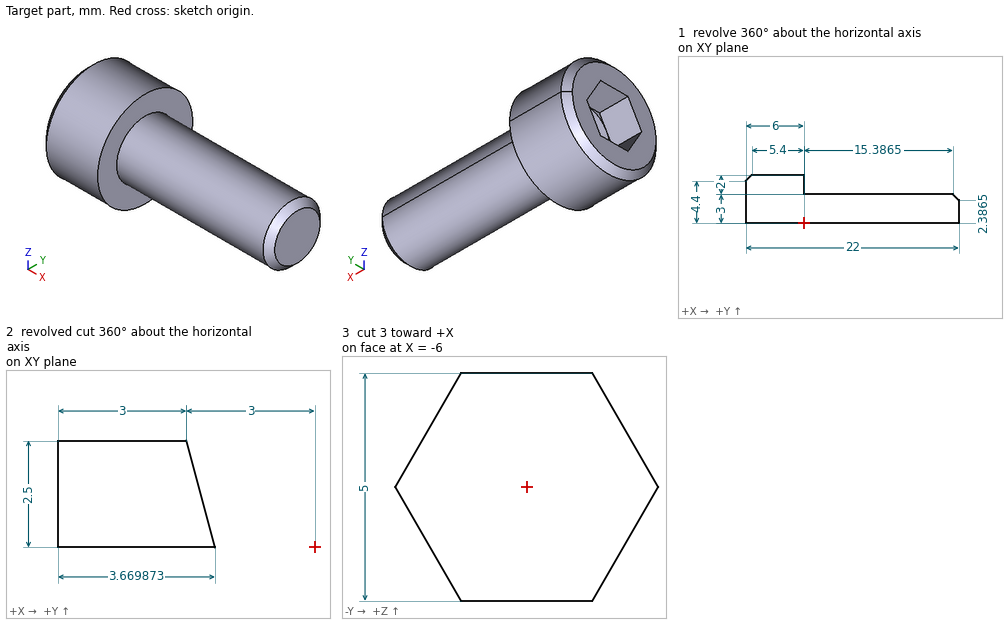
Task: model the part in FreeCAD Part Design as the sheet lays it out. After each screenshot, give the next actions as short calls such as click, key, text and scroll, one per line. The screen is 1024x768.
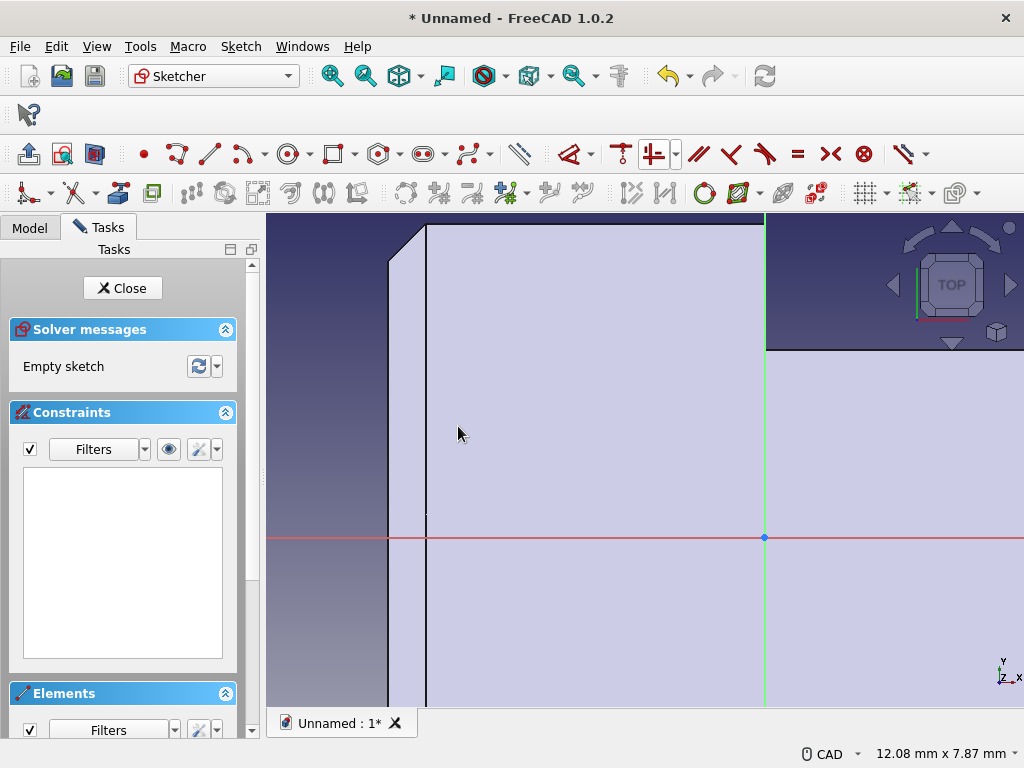
click(177, 154)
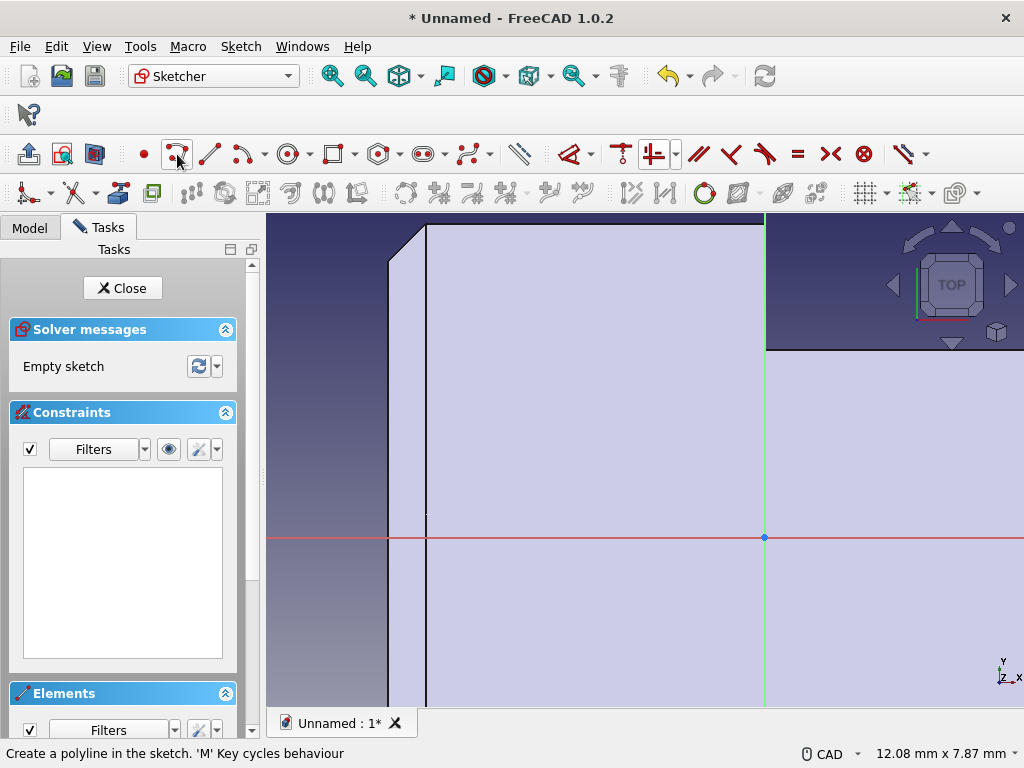
click(618, 538)
click(576, 381)
click(388, 381)
click(388, 529)
click(618, 538)
key(Escape)
key(Escape)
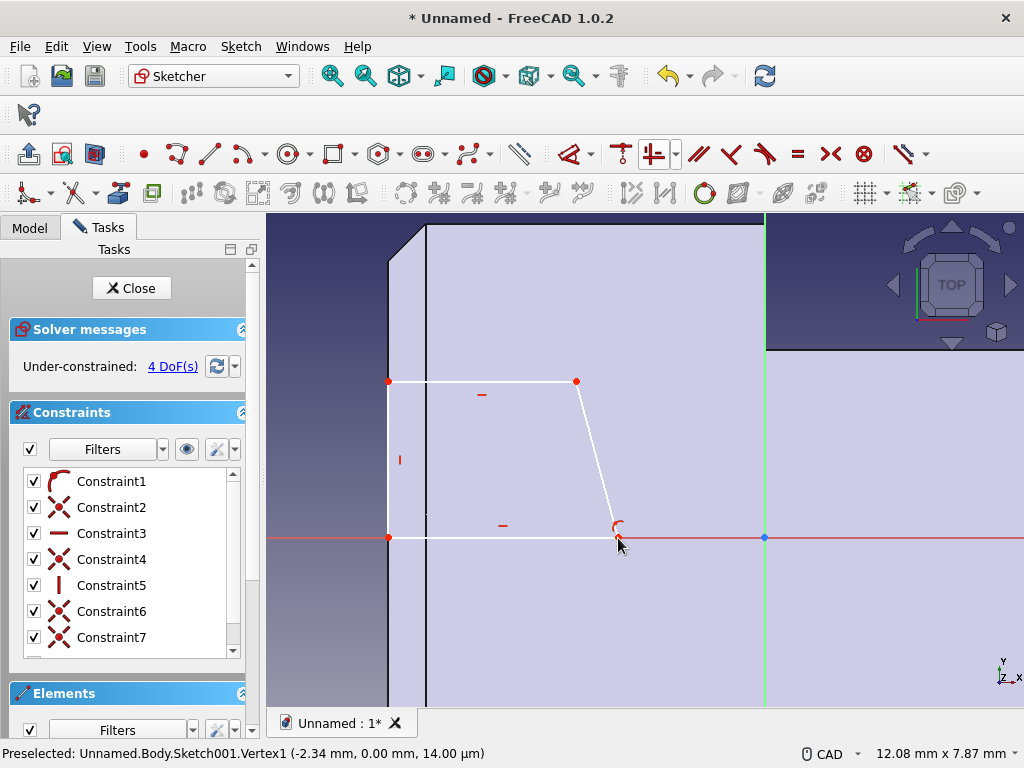
click(568, 154)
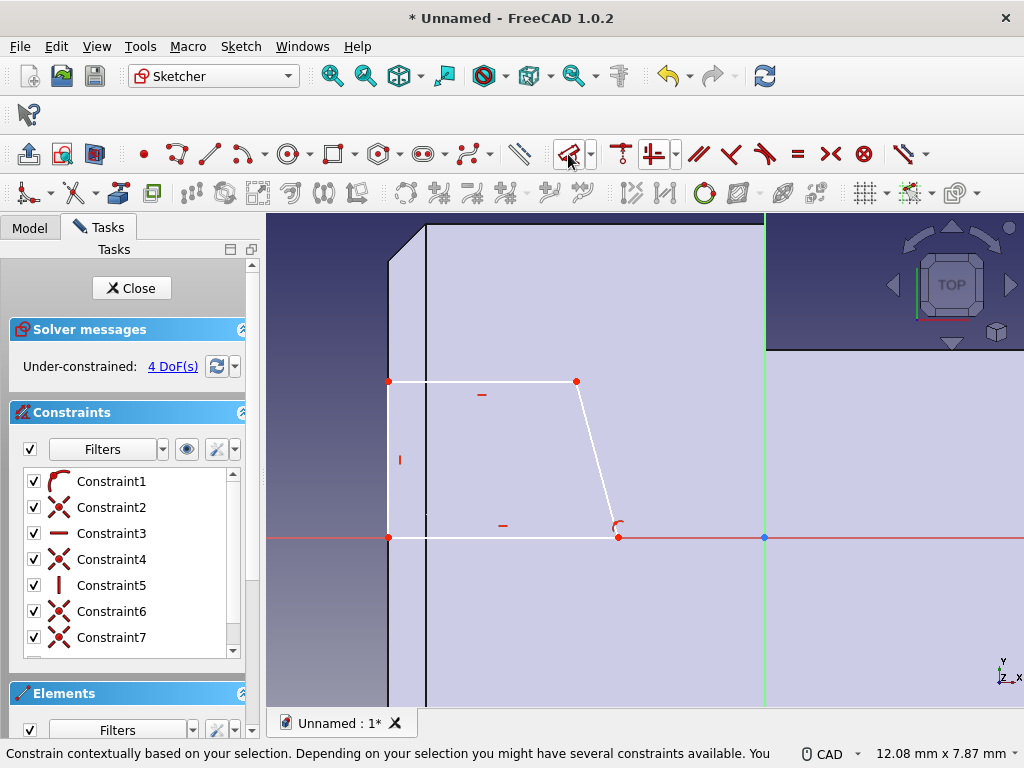
click(520, 382)
click(482, 348)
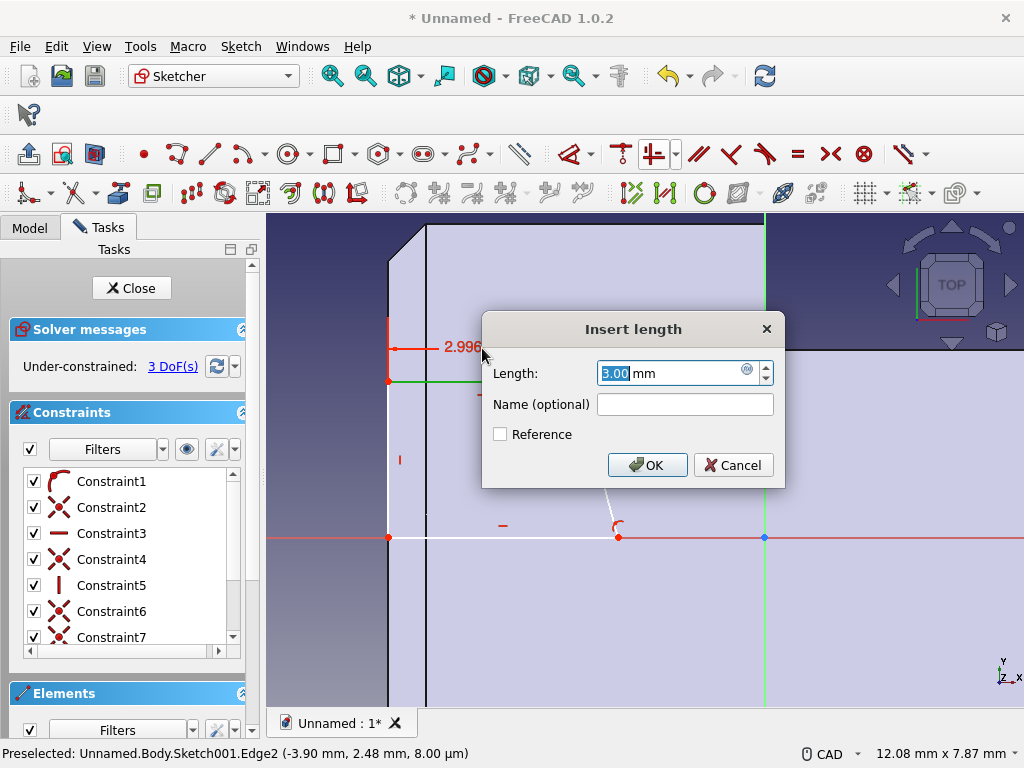
text(3)
key(Return)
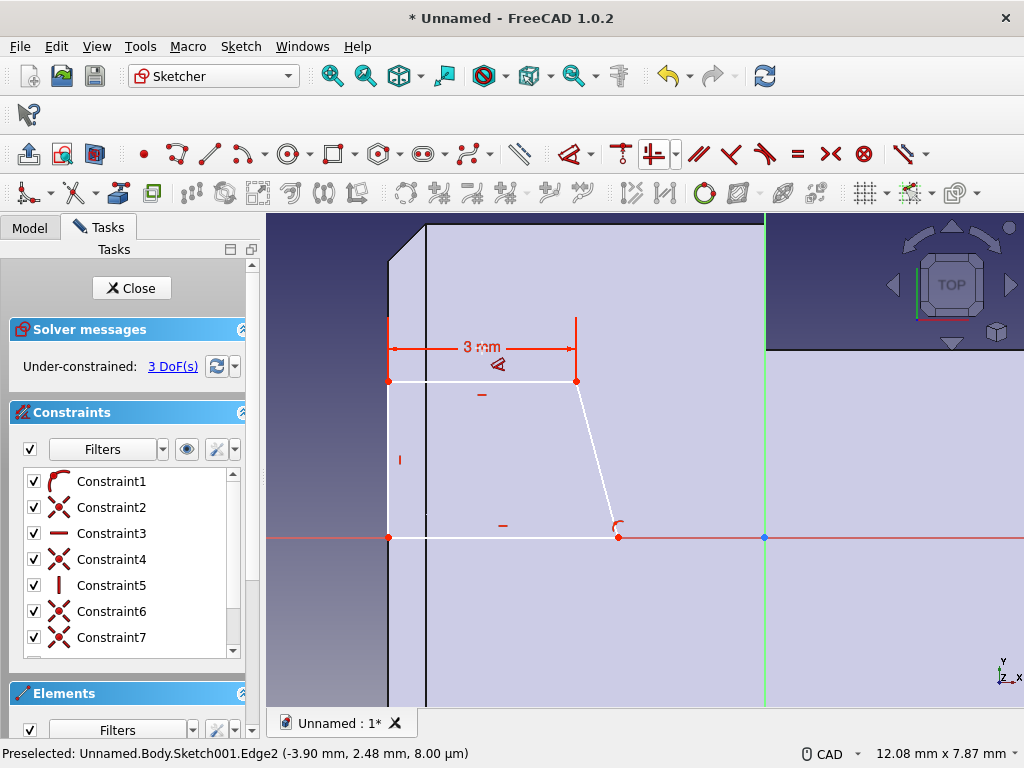
click(576, 382)
click(670, 572)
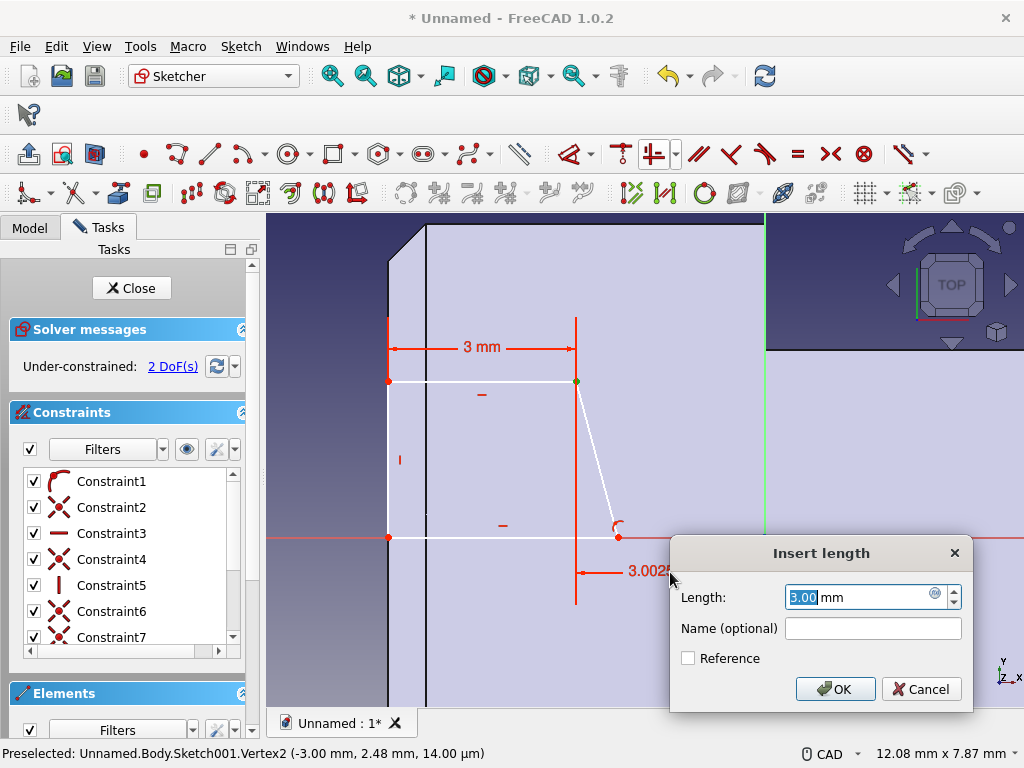
text(3)
key(Return)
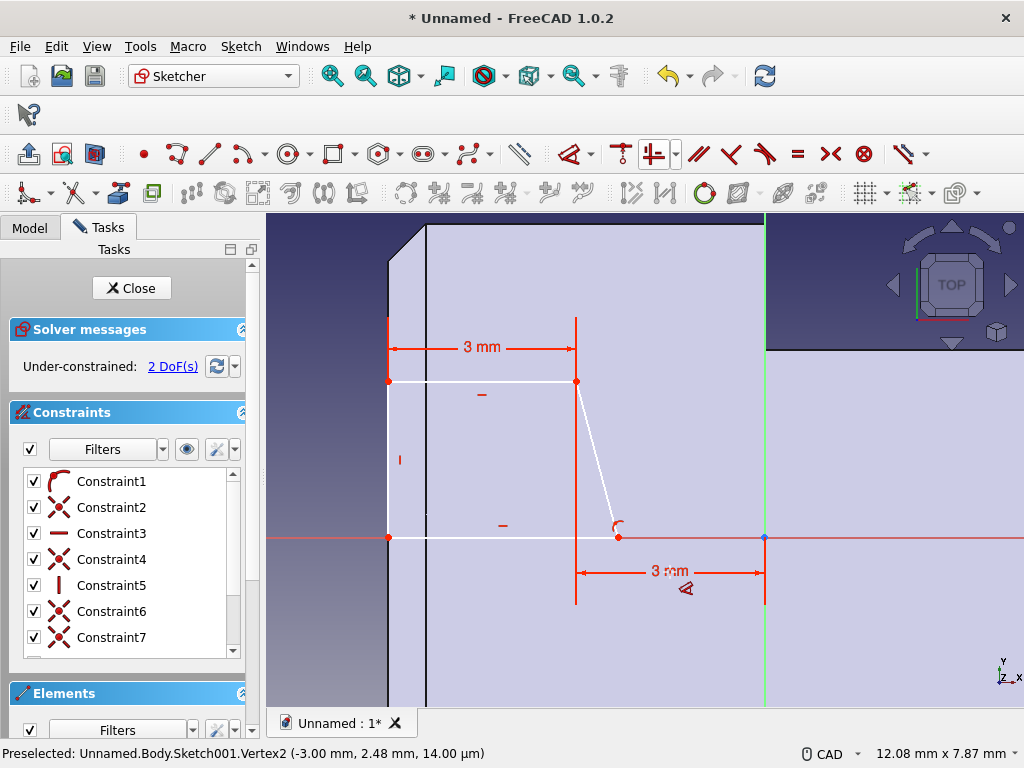
click(388, 429)
click(354, 460)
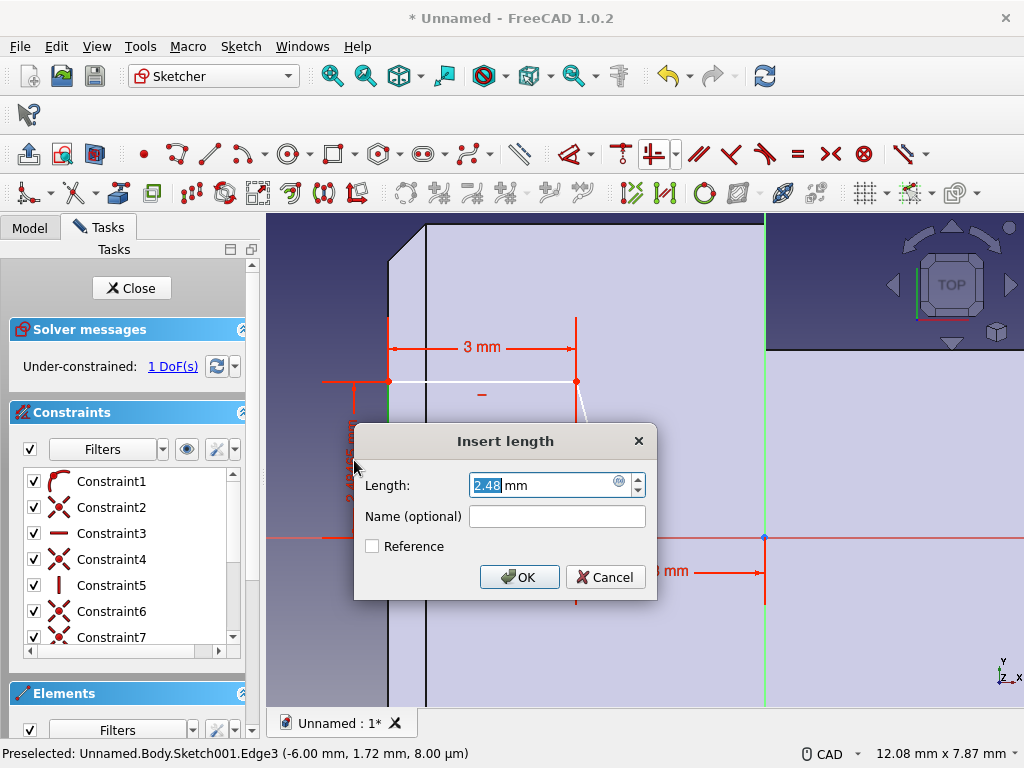
text(2.5)
key(Return)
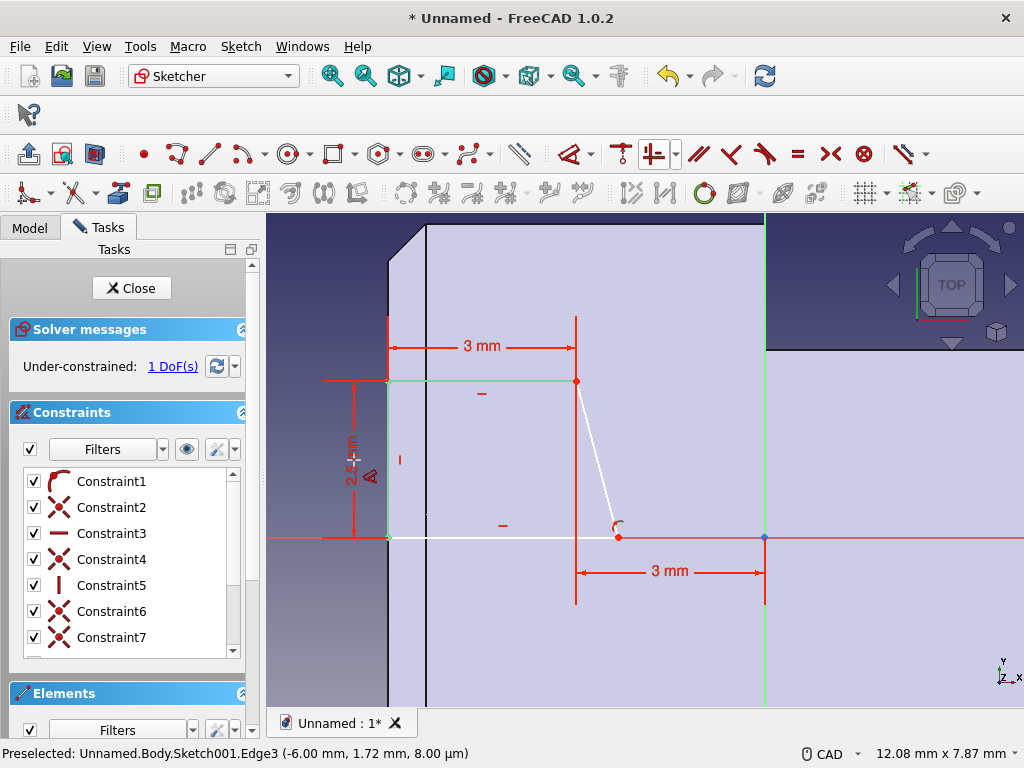
click(457, 538)
click(503, 572)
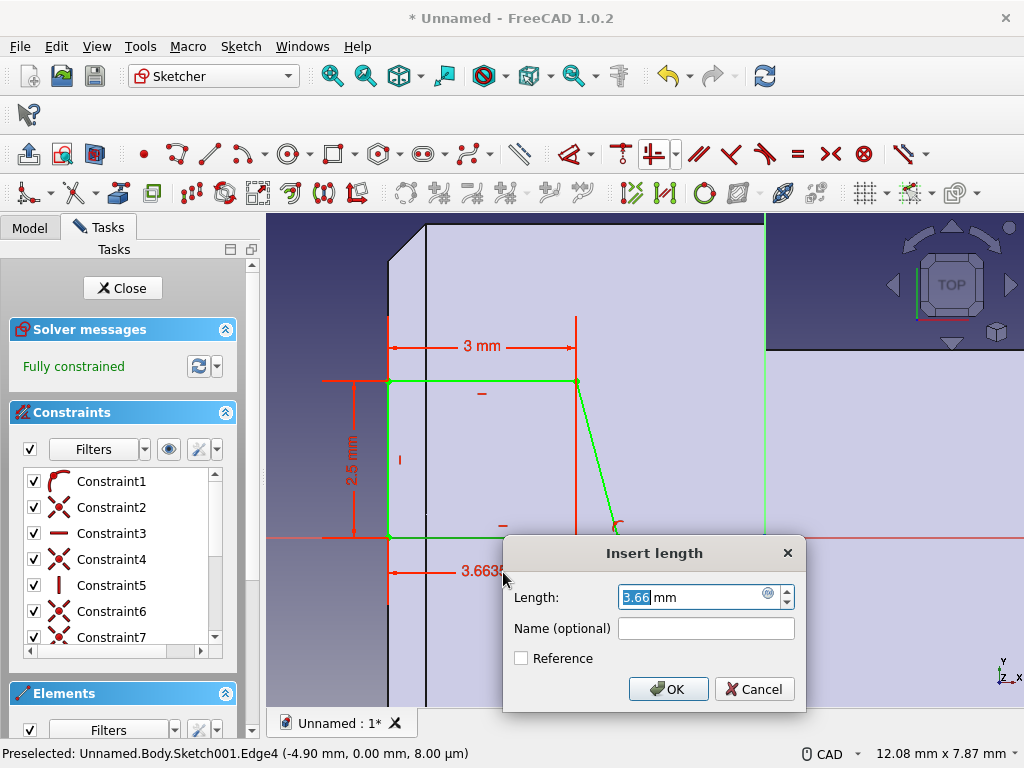
text(3.669873)
key(Return)
key(Escape)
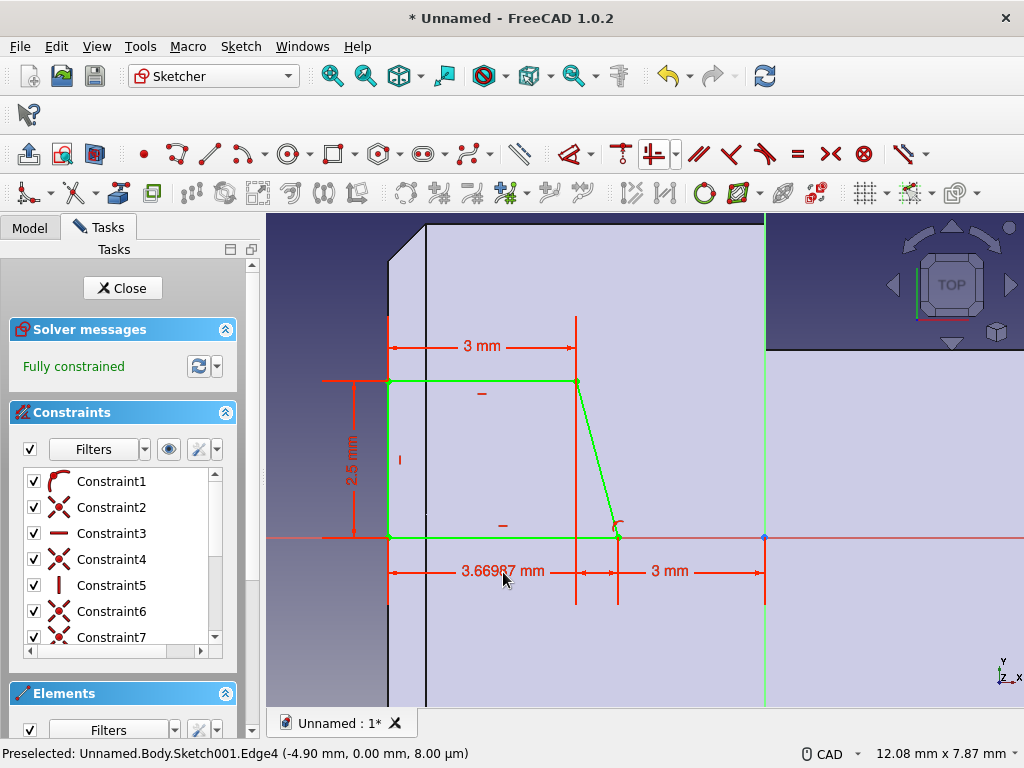
click(123, 288)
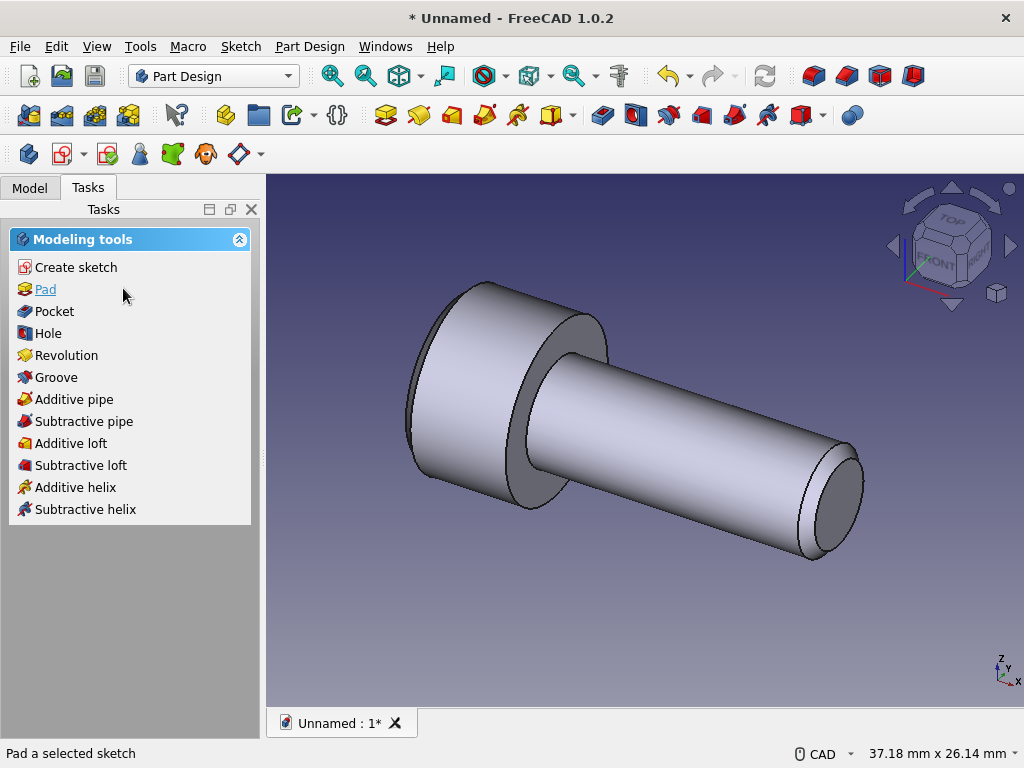
click(669, 116)